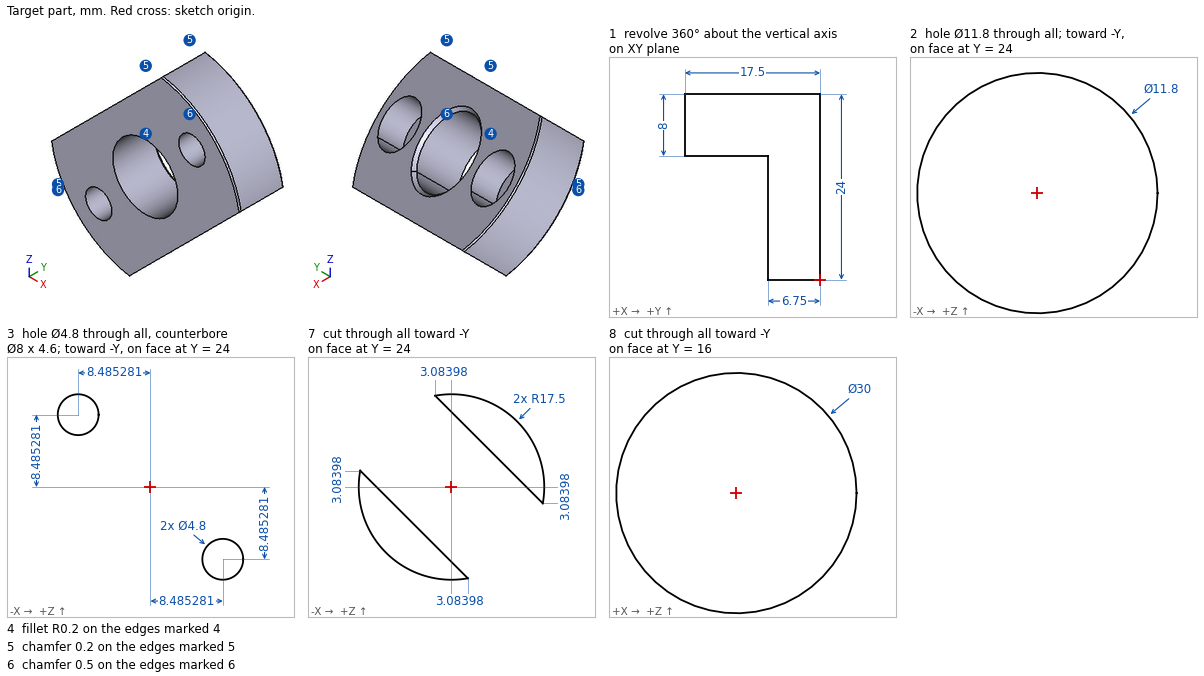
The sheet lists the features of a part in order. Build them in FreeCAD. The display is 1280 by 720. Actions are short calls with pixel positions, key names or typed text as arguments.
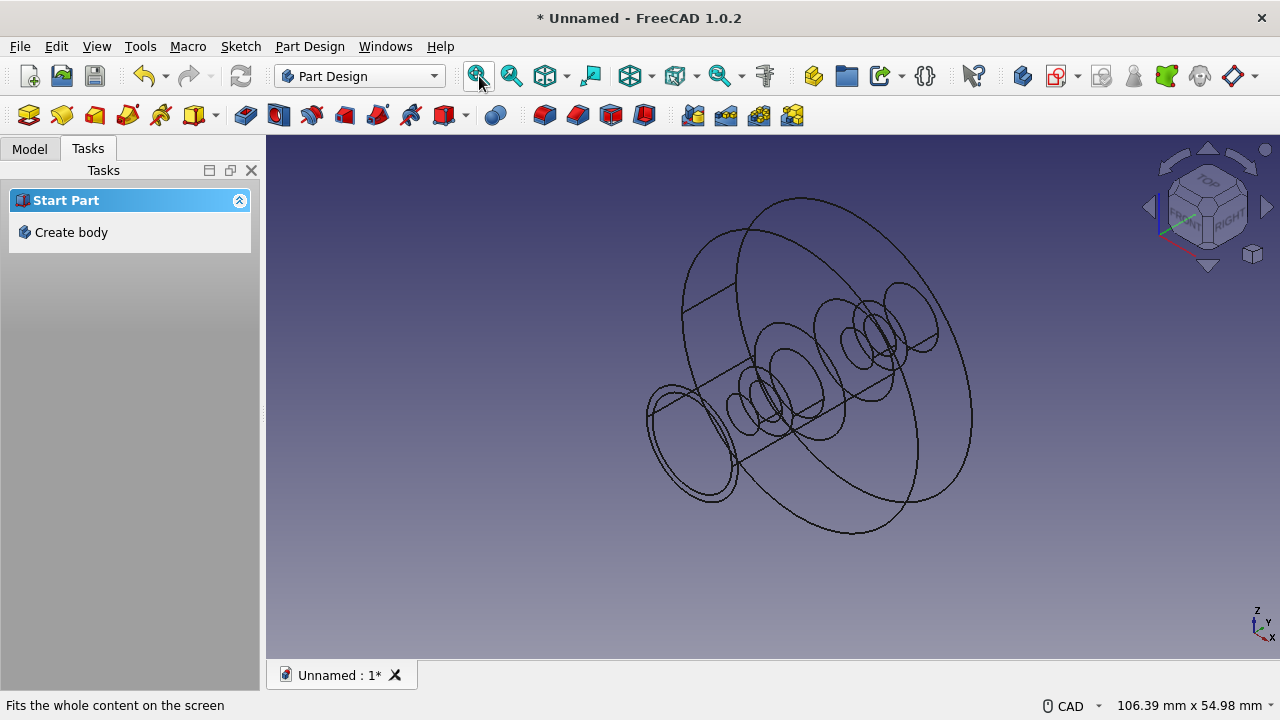
click(846, 407)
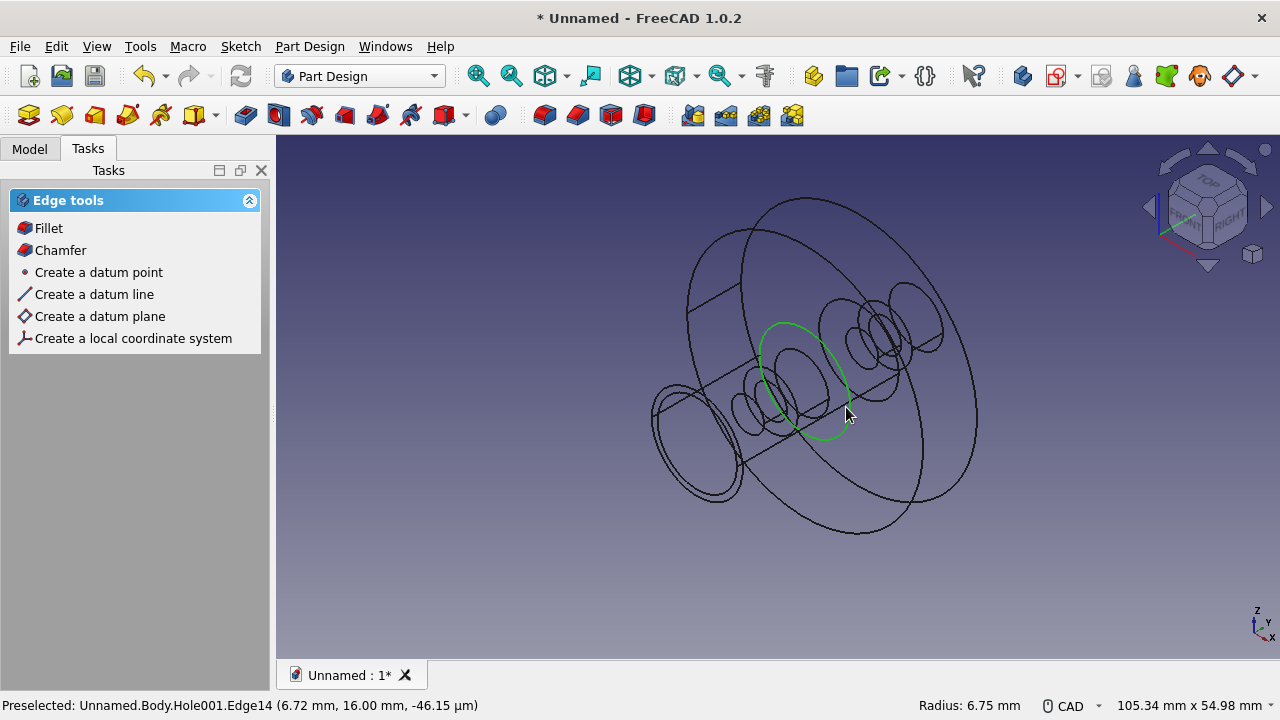
key(v)
key(1)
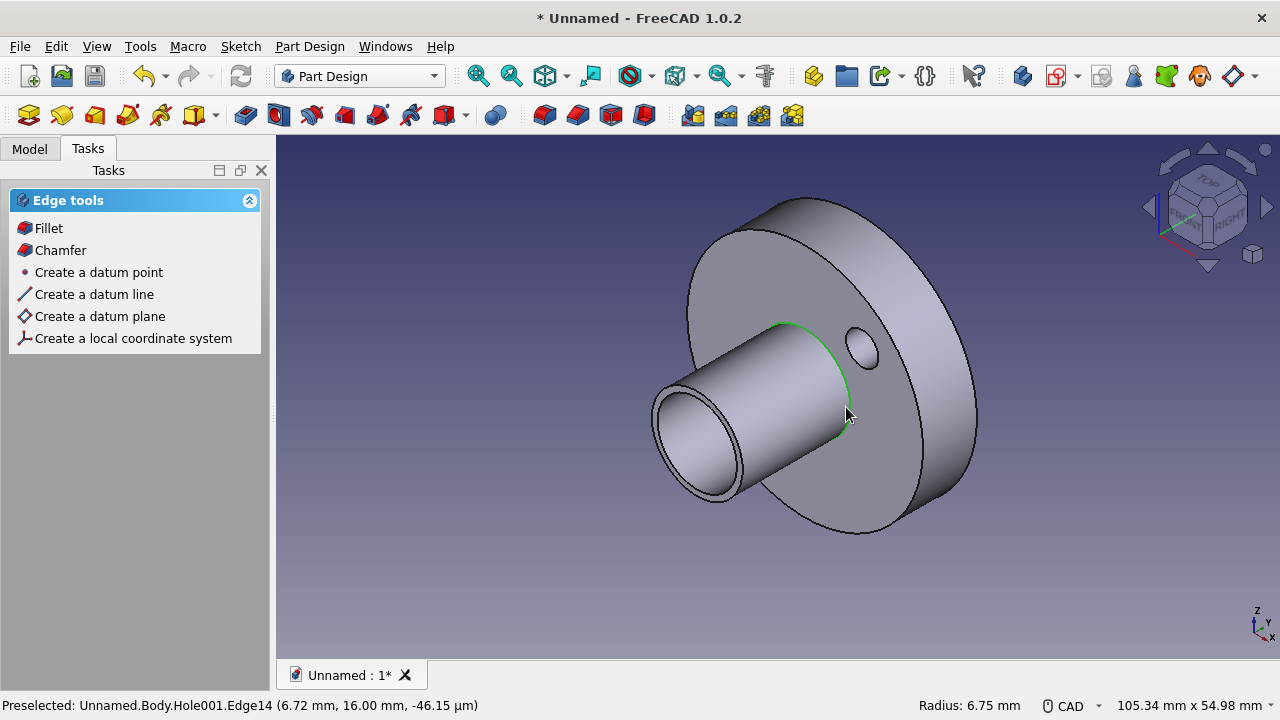
click(545, 116)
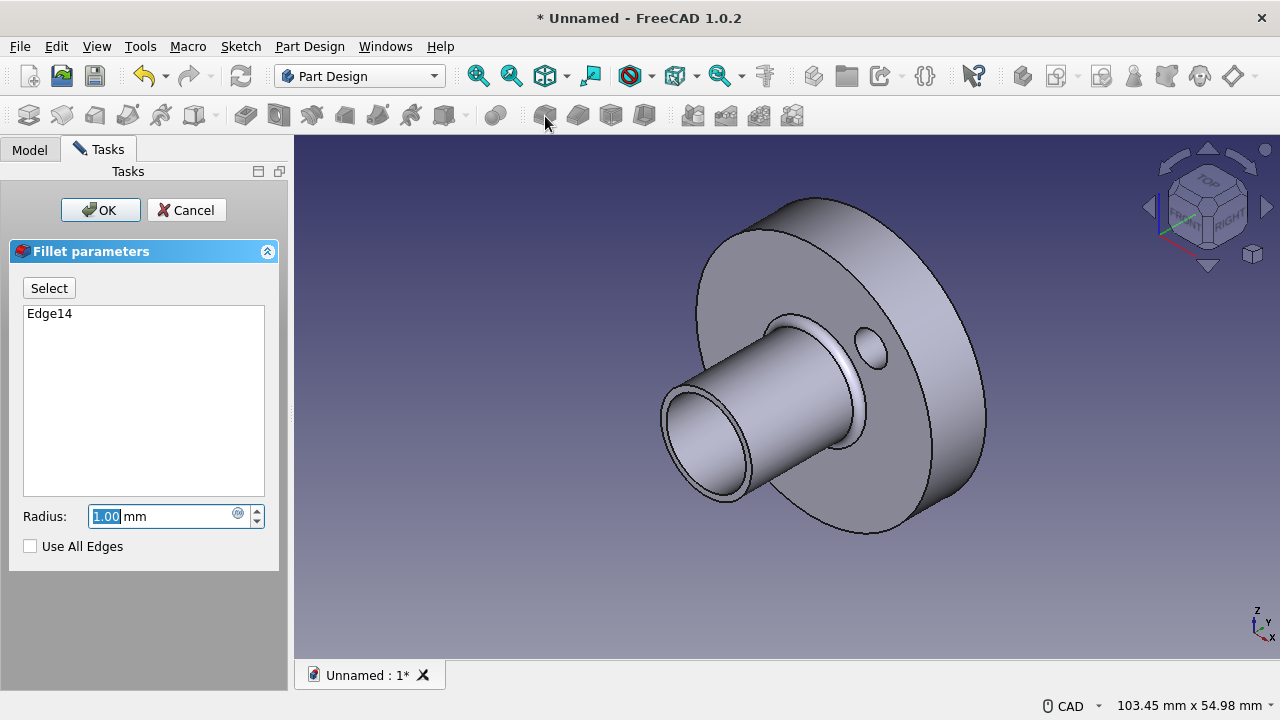
text(0.2)
key(Tab)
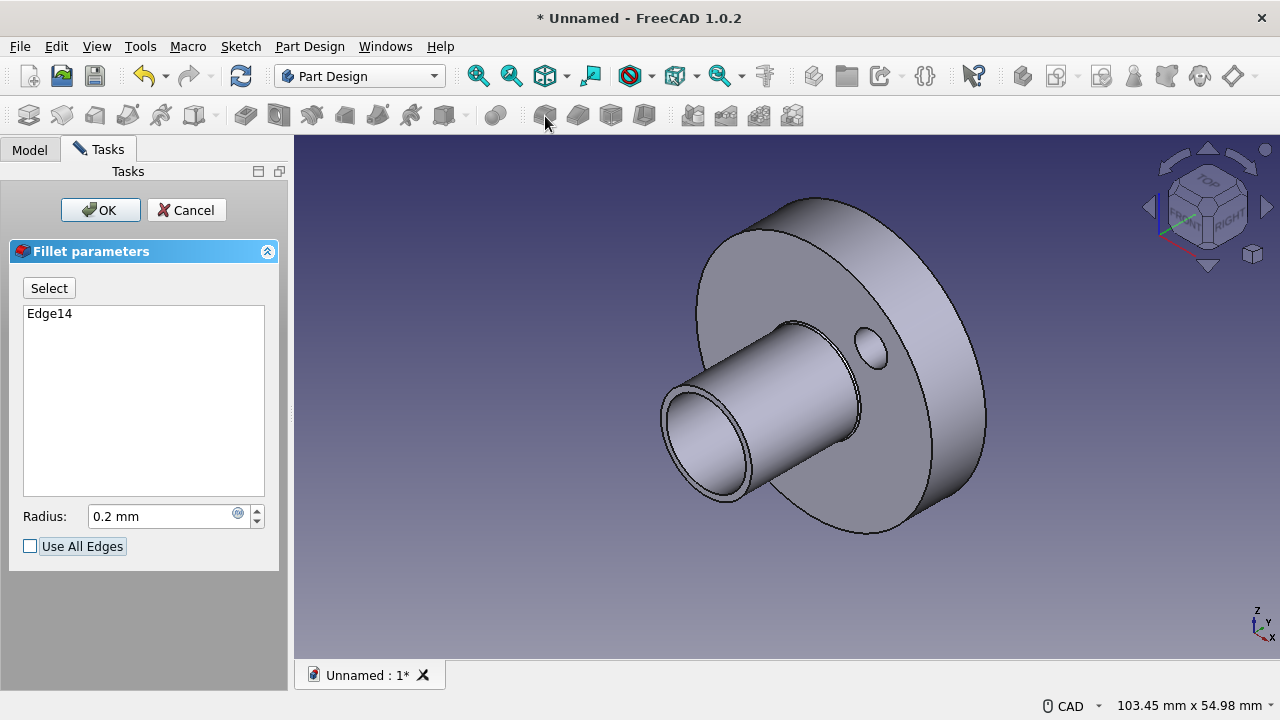
click(101, 210)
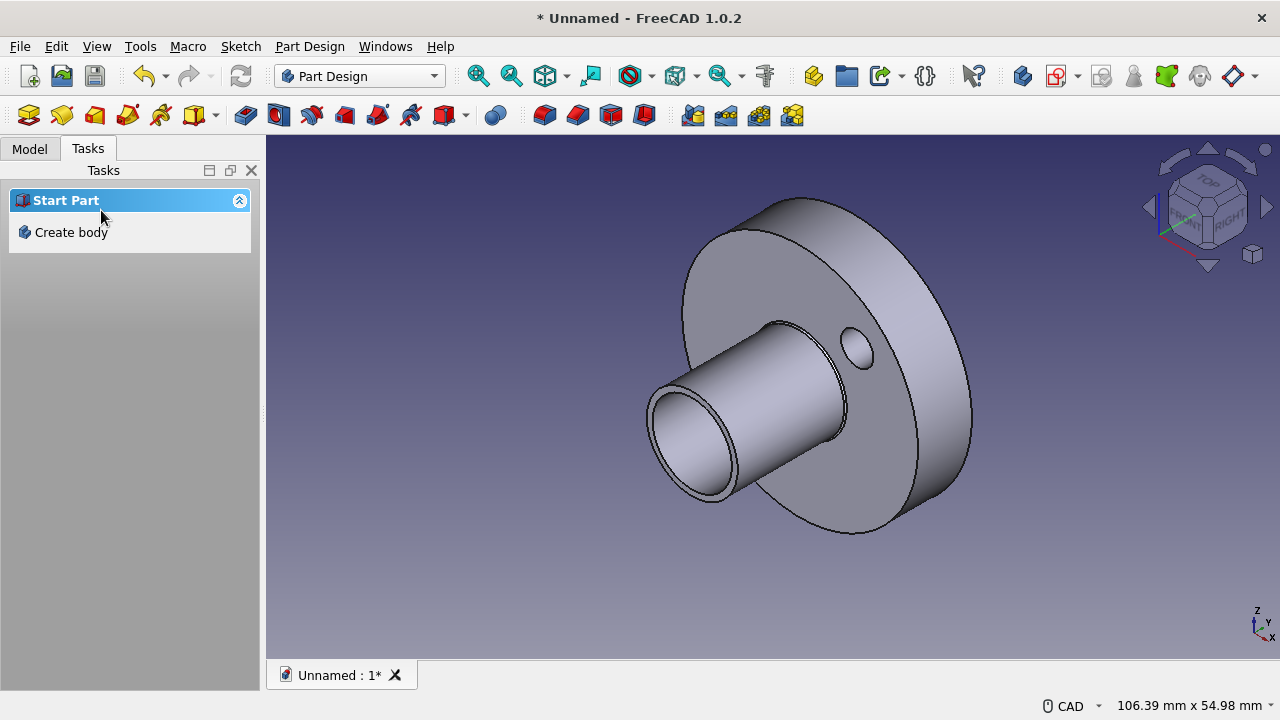
click(738, 469)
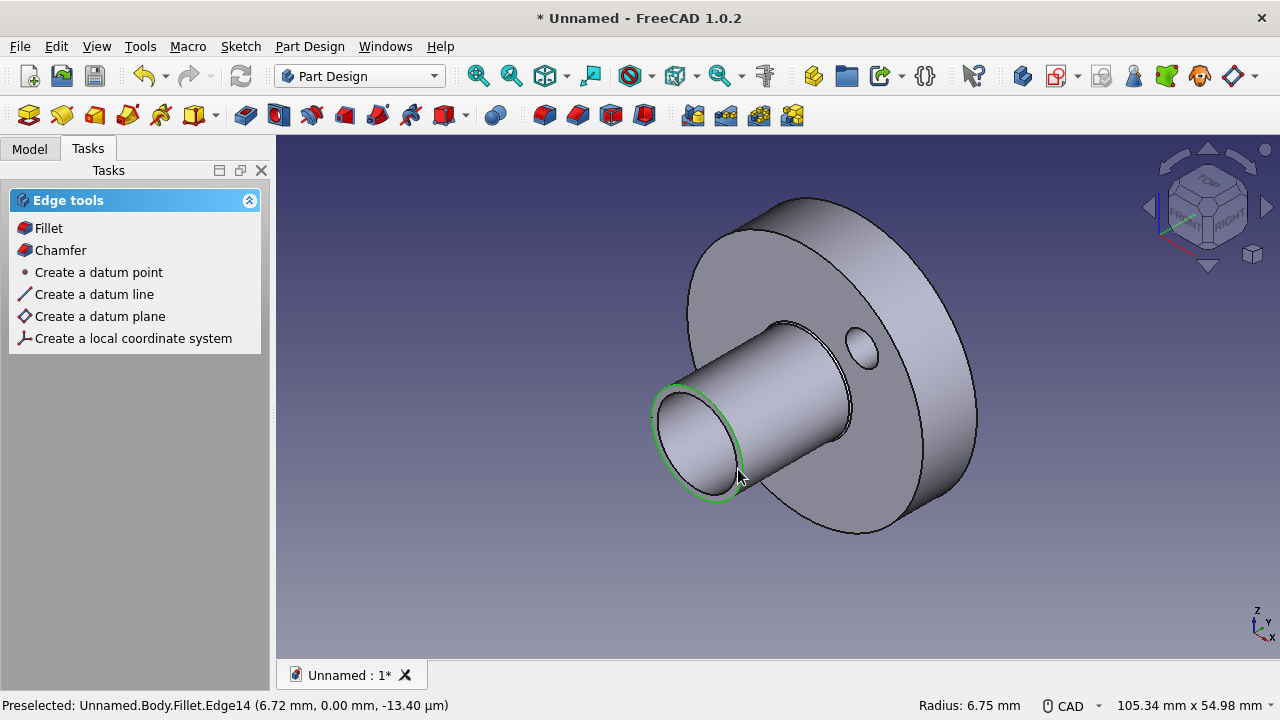
click(923, 449, ctrl)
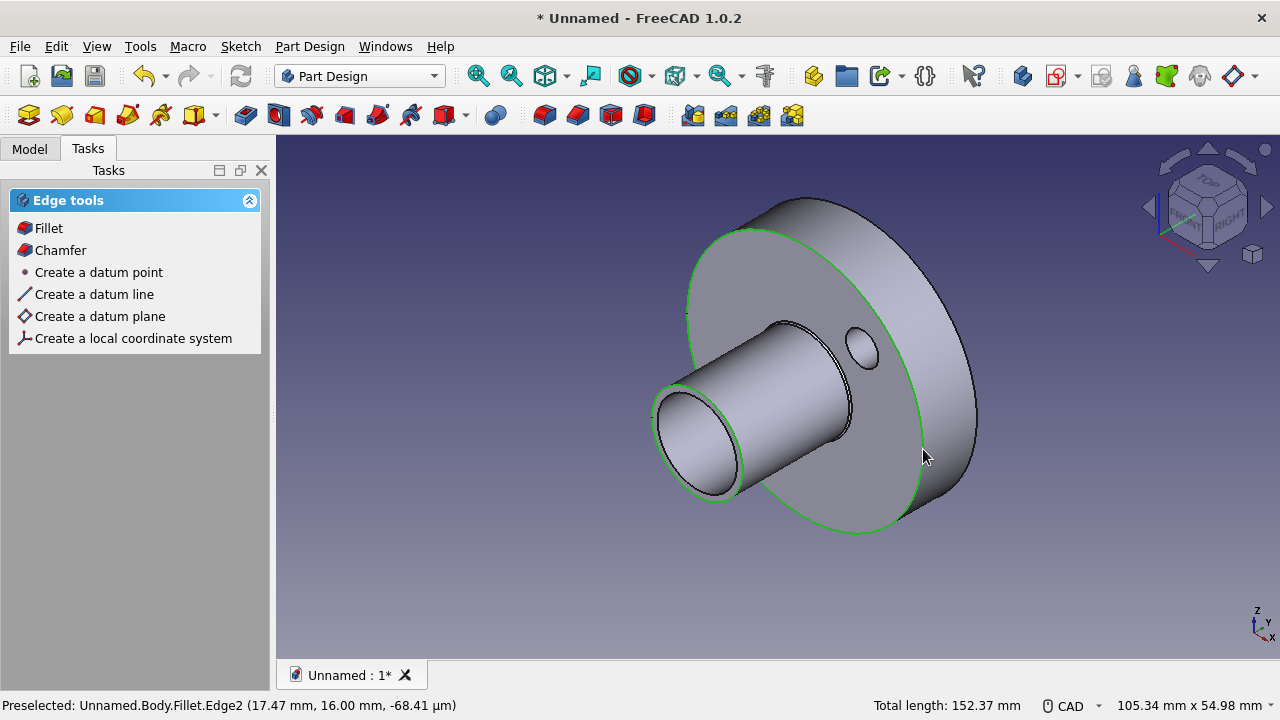
key(2)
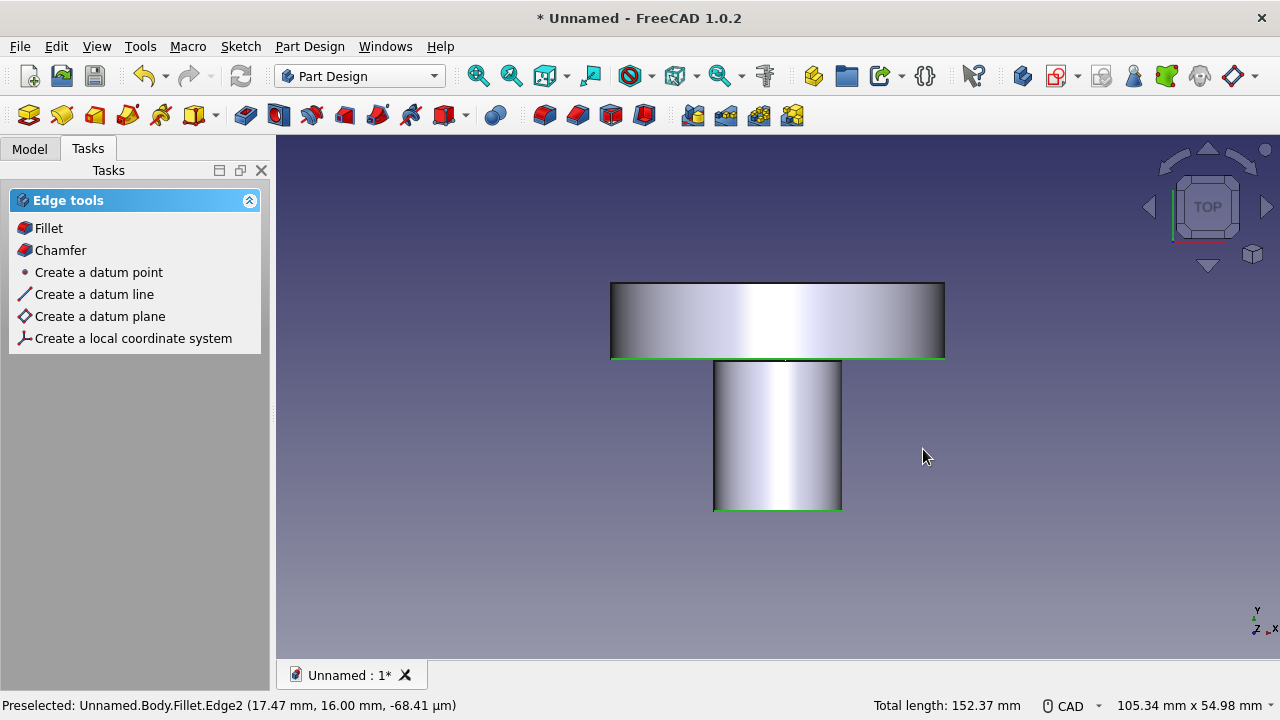
key(v)
key(f)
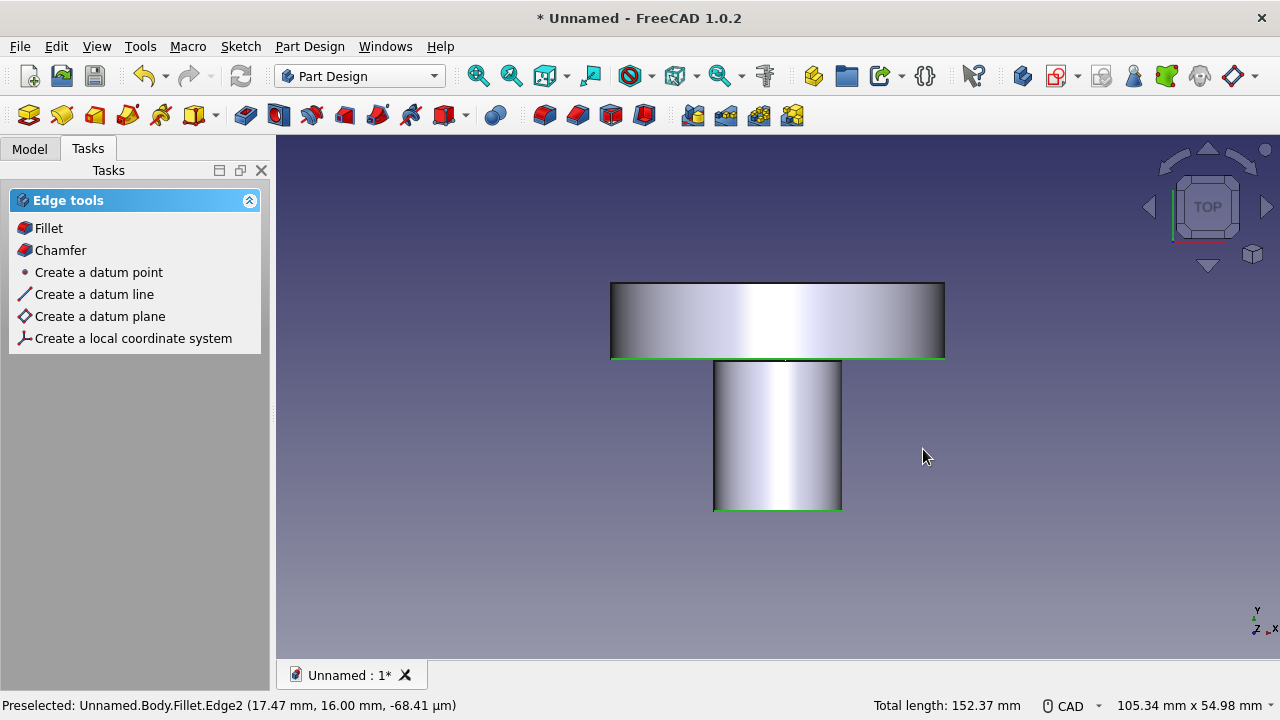
click(913, 282, ctrl)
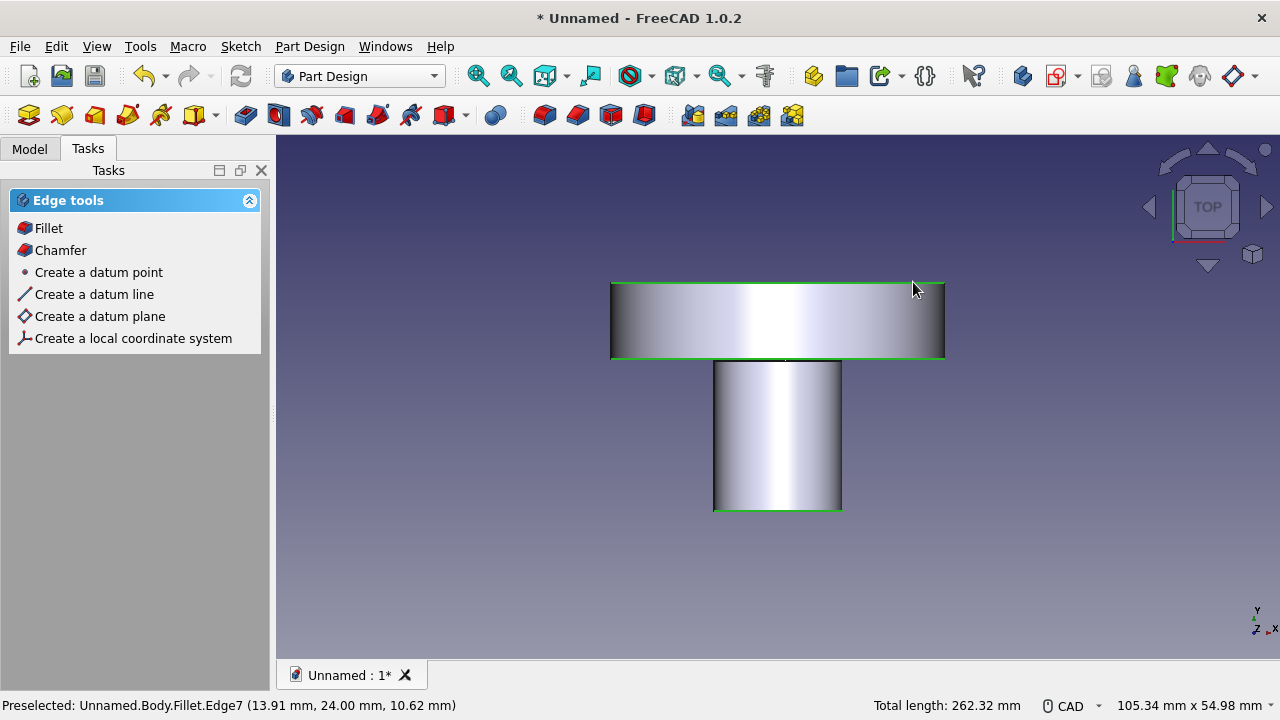
click(578, 116)